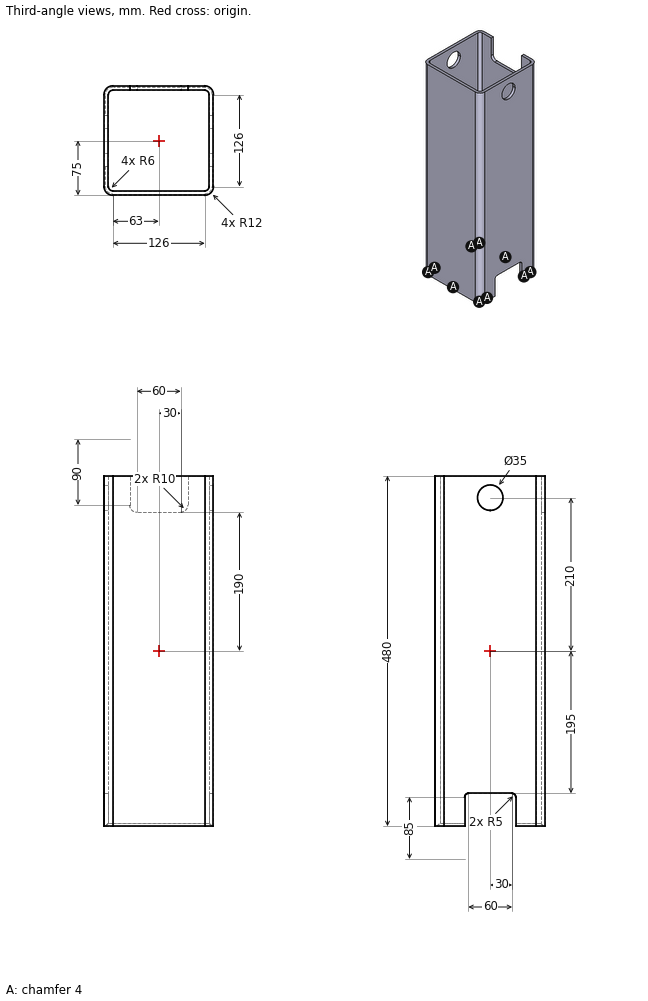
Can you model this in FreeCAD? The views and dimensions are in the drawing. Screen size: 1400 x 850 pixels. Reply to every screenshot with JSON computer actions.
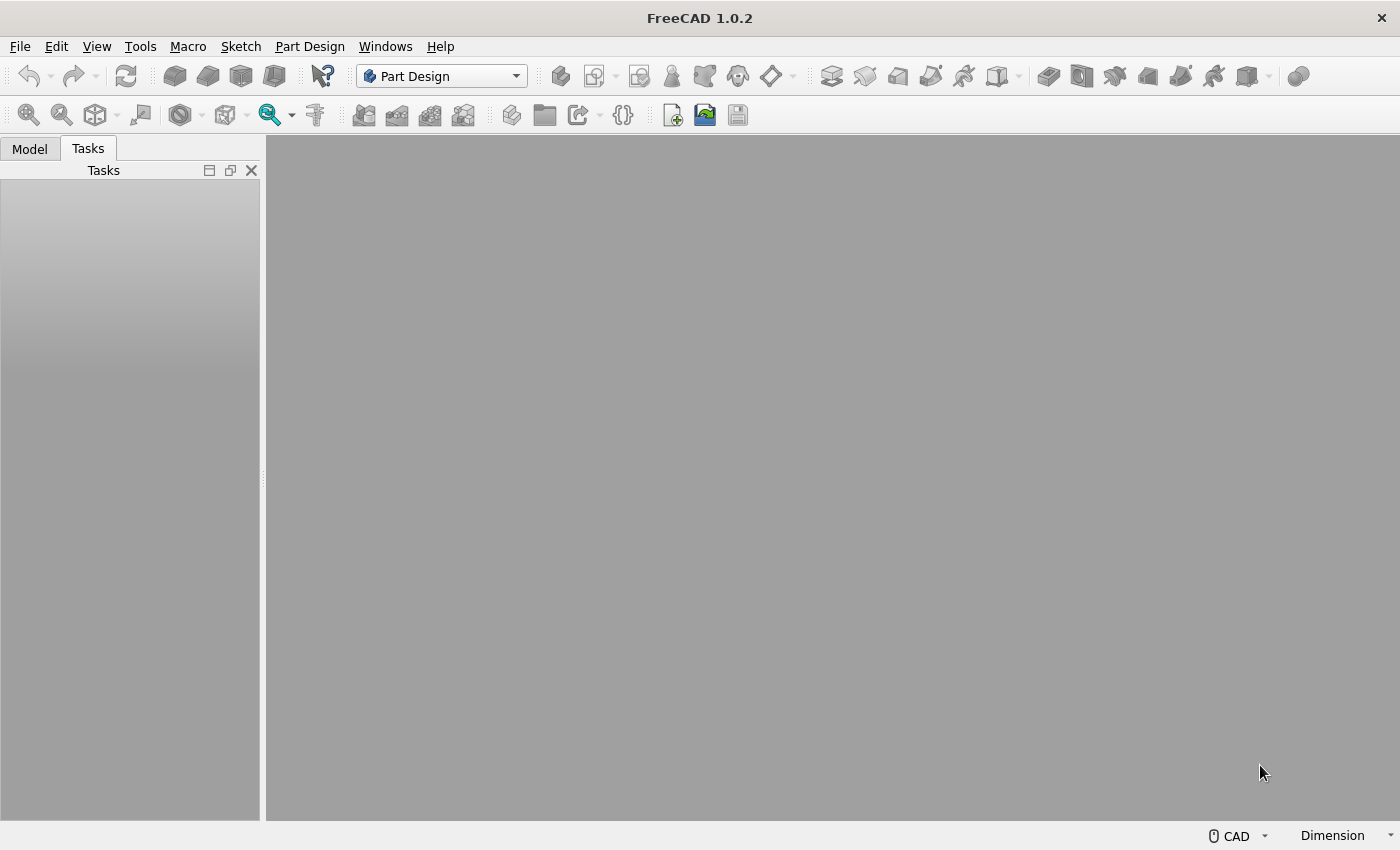
{"action": "key", "text": "ctrl+n"}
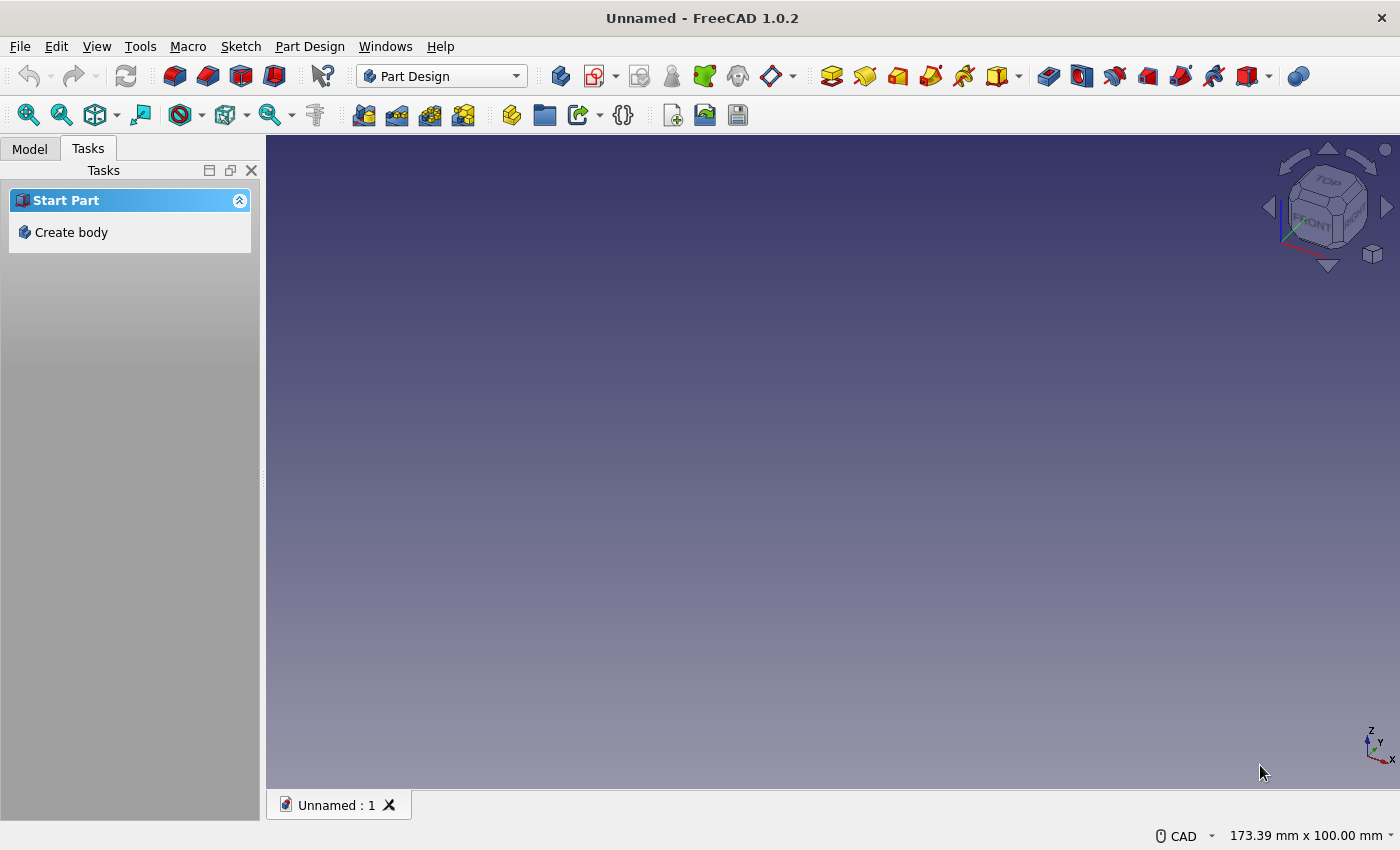
{"action": "left_click", "coordinate": [594, 76]}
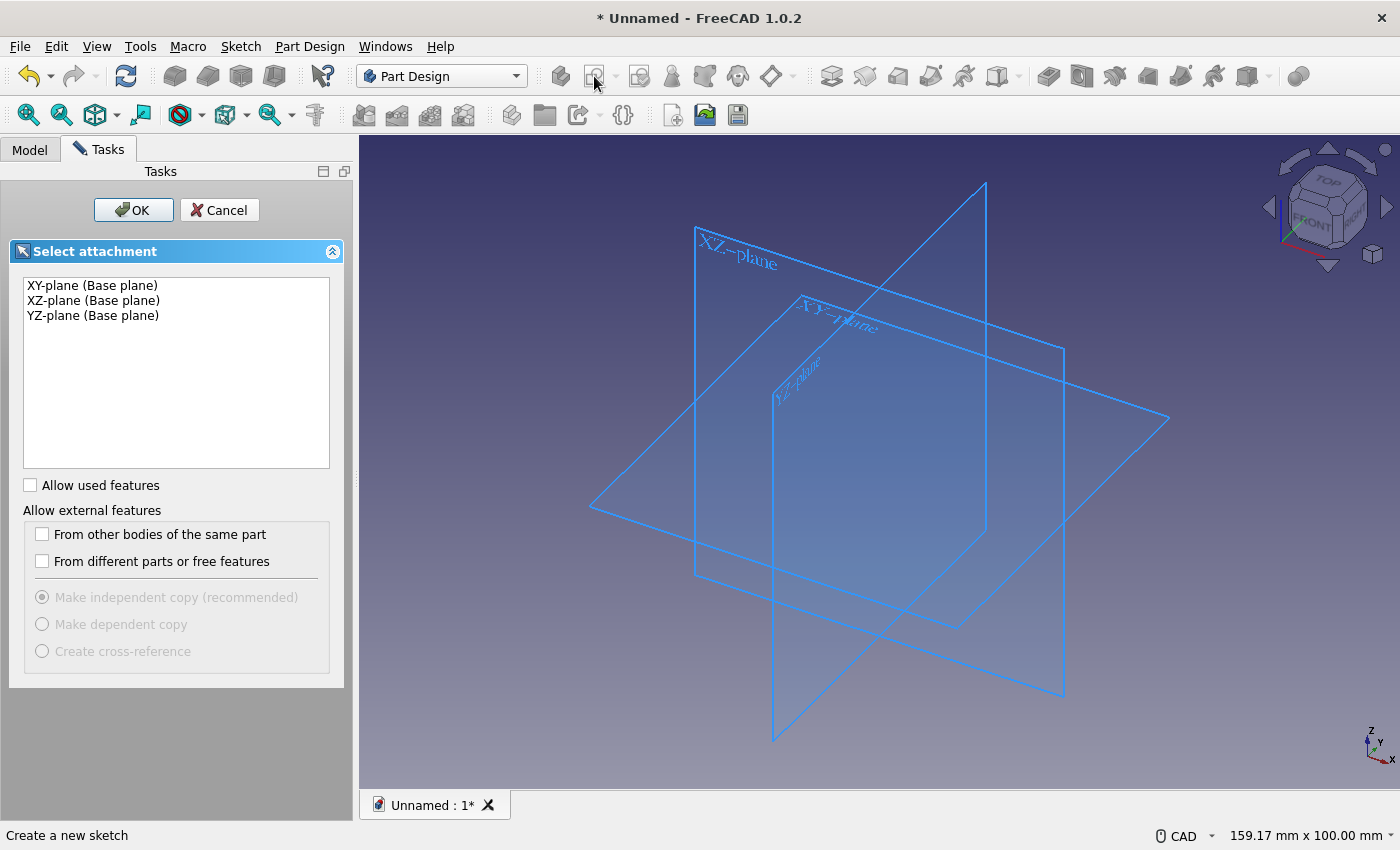
{"action": "left_click", "coordinate": [84, 286]}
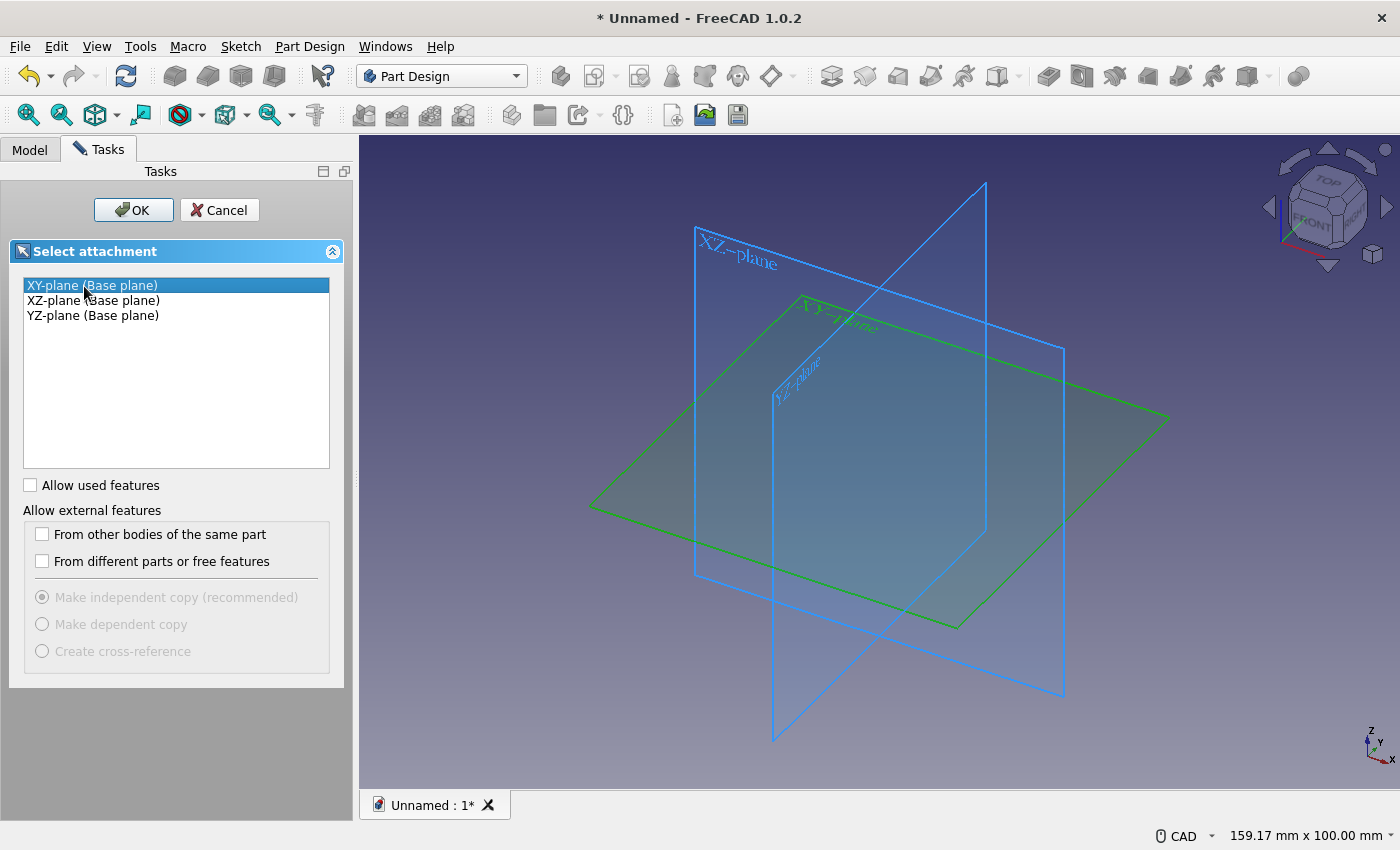
{"action": "left_click", "coordinate": [134, 210]}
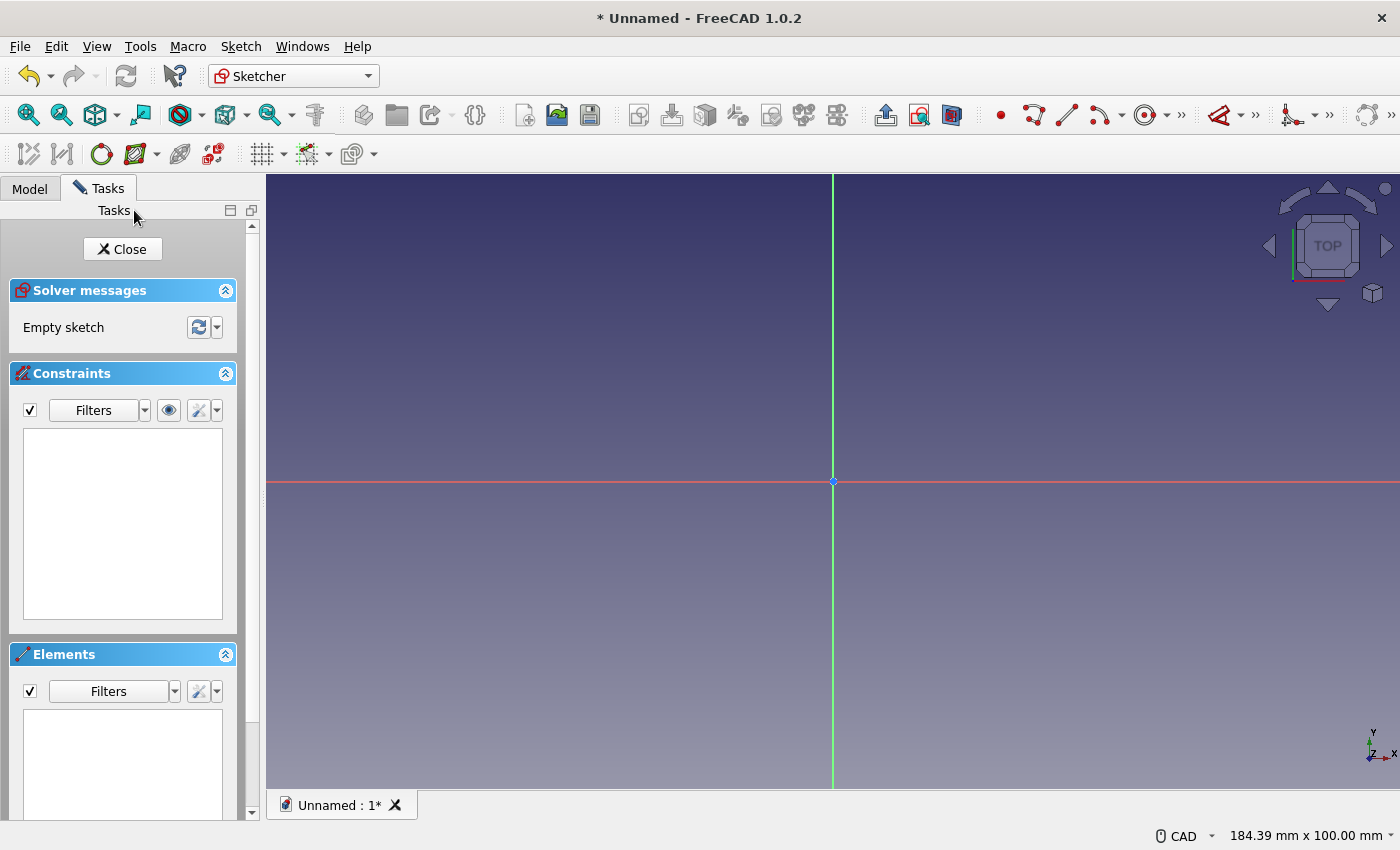
{"action": "scroll", "coordinate": [709, 482], "scroll_direction": "down", "scroll_amount": 4}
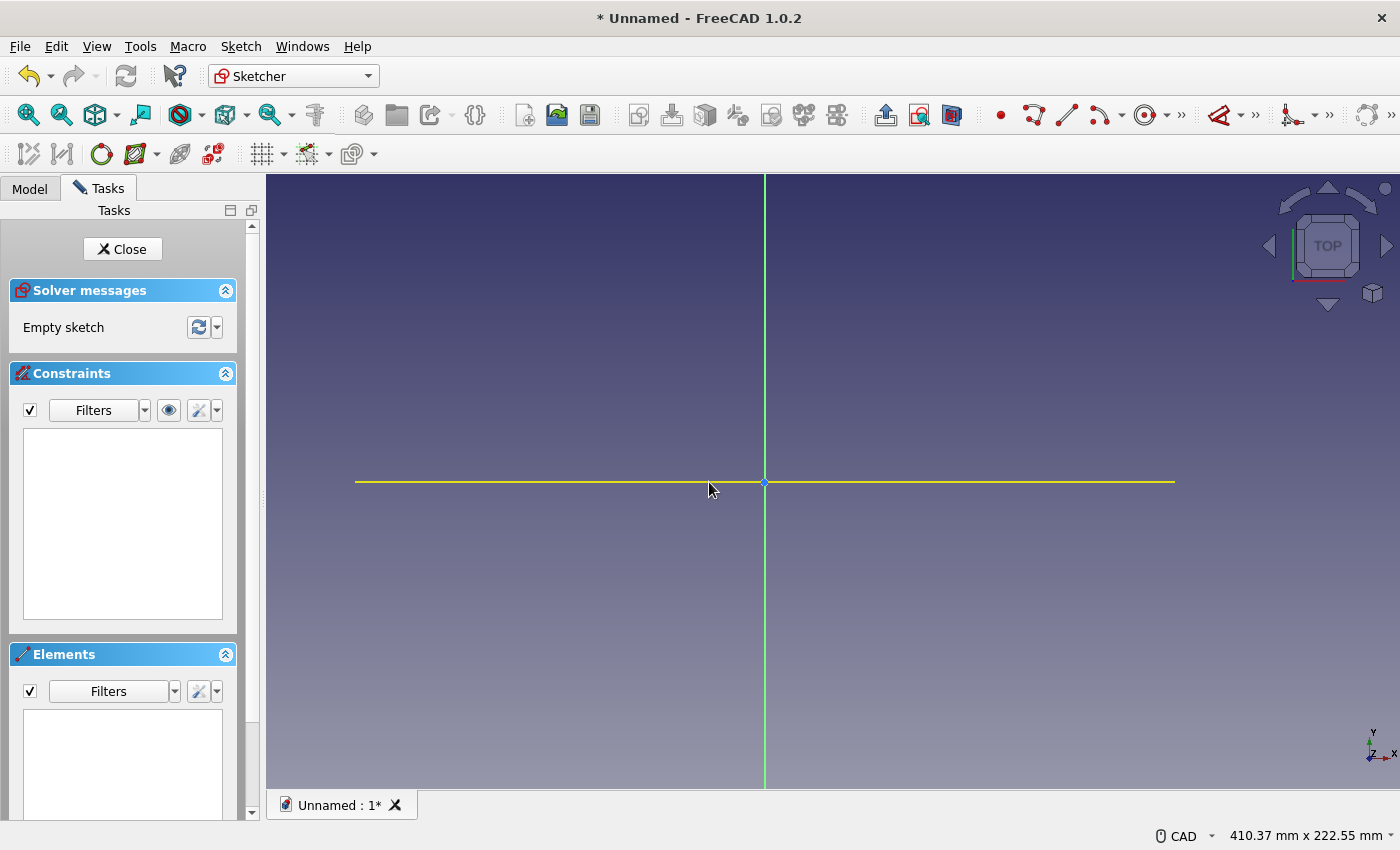
{"action": "key", "text": "g l"}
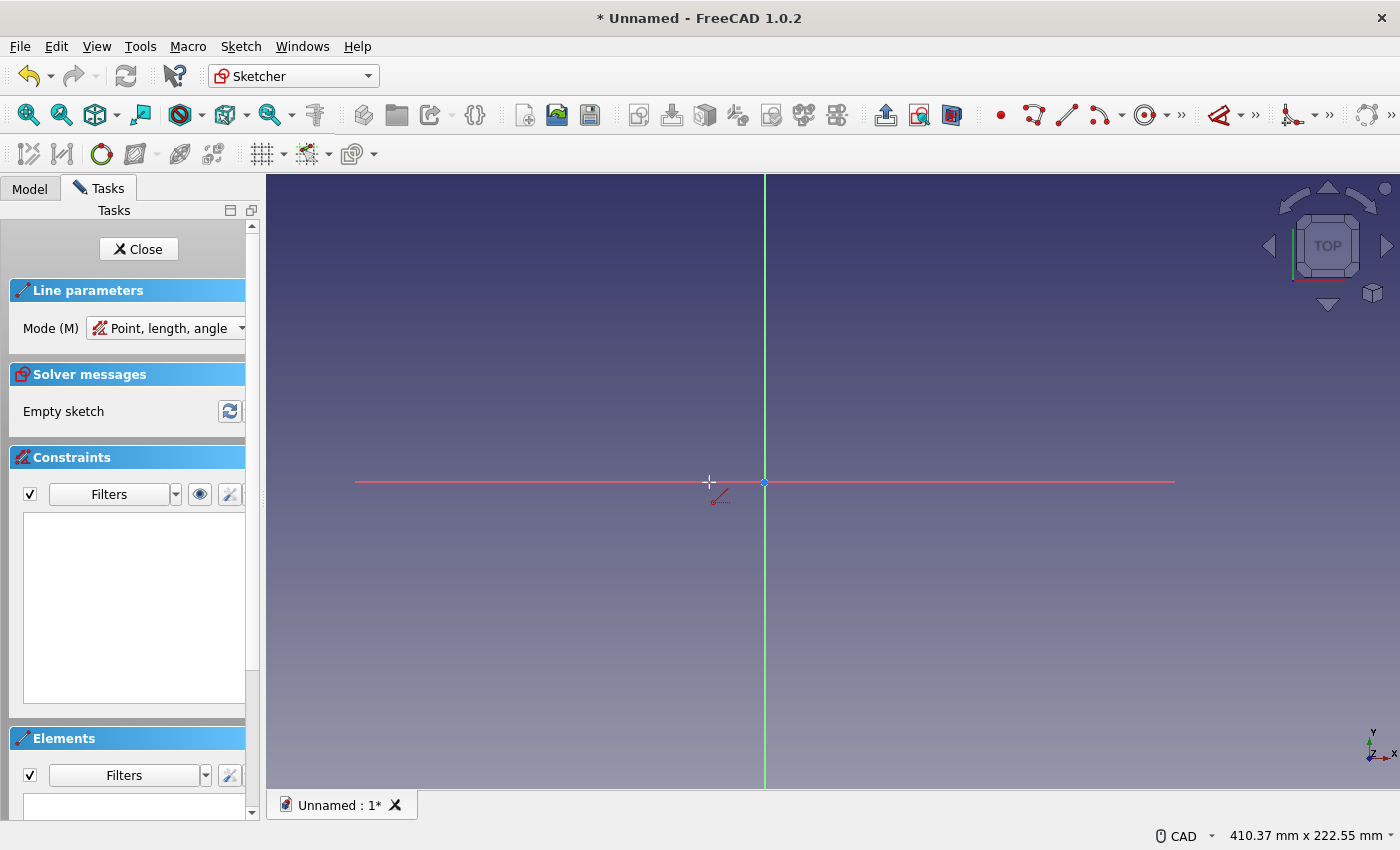
{"action": "left_click", "coordinate": [591, 689]}
{"action": "left_click", "coordinate": [939, 689]}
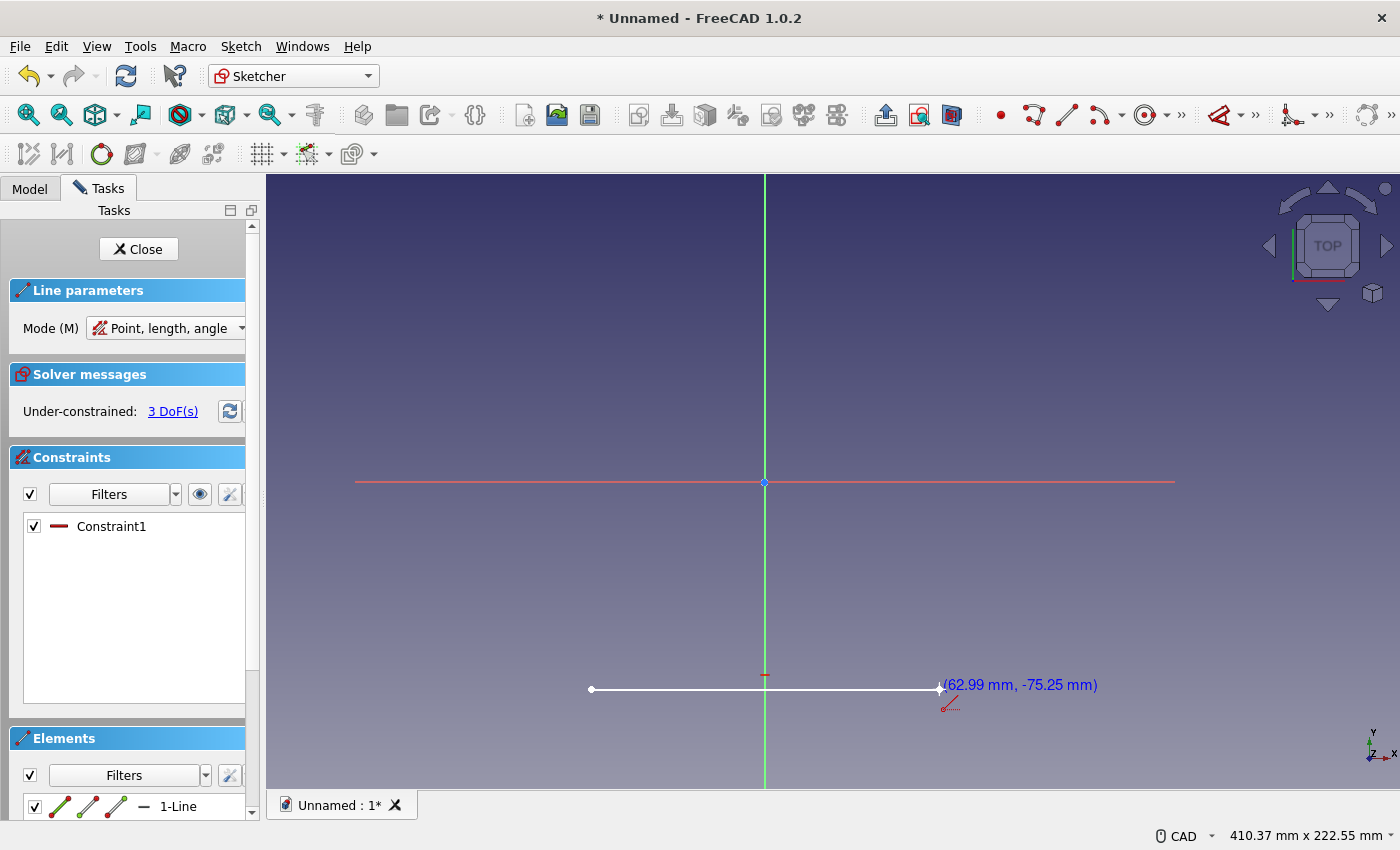
{"action": "left_click", "coordinate": [972, 656]}
{"action": "left_click", "coordinate": [972, 308]}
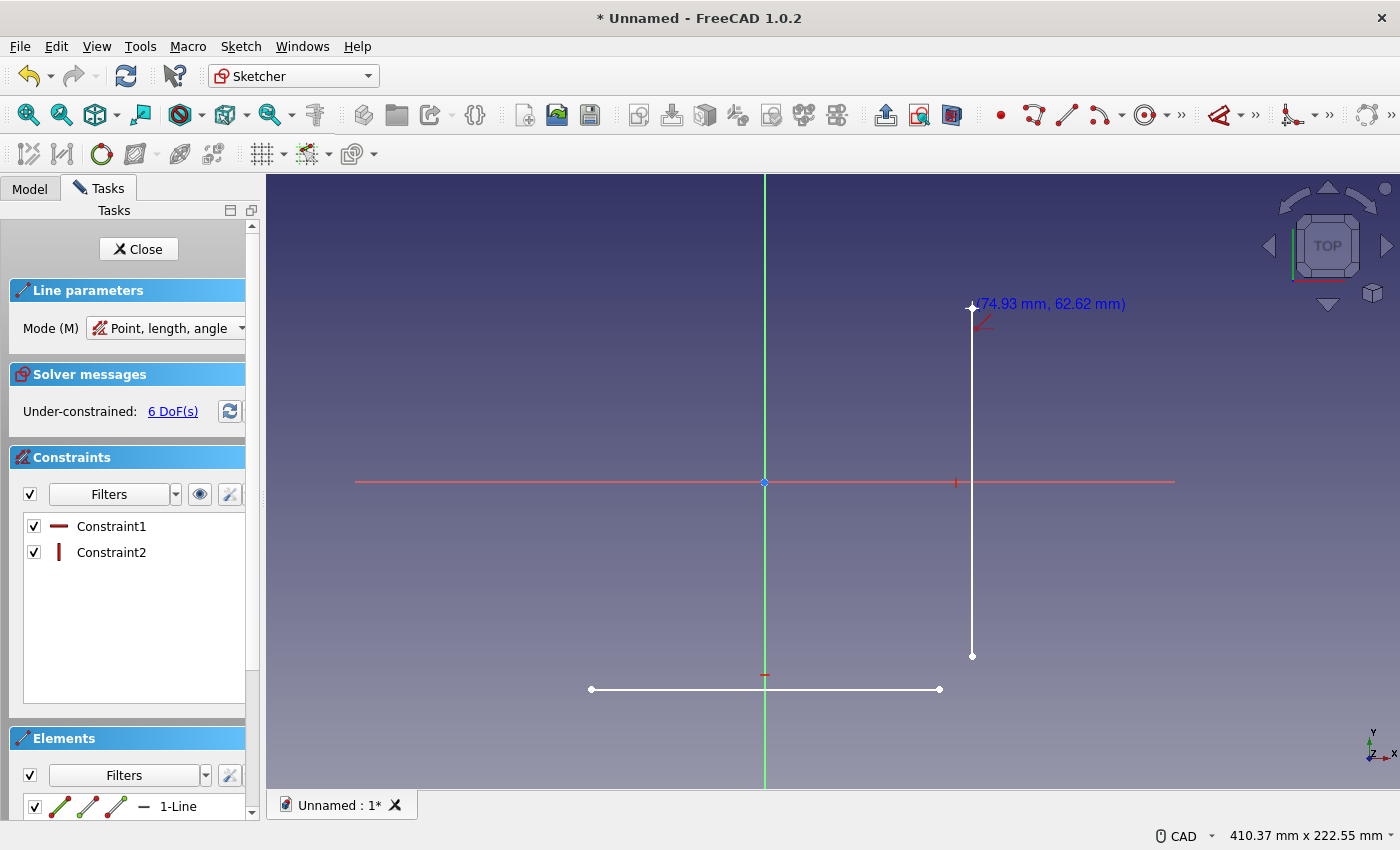
{"action": "left_click", "coordinate": [939, 275]}
{"action": "left_click", "coordinate": [591, 275]}